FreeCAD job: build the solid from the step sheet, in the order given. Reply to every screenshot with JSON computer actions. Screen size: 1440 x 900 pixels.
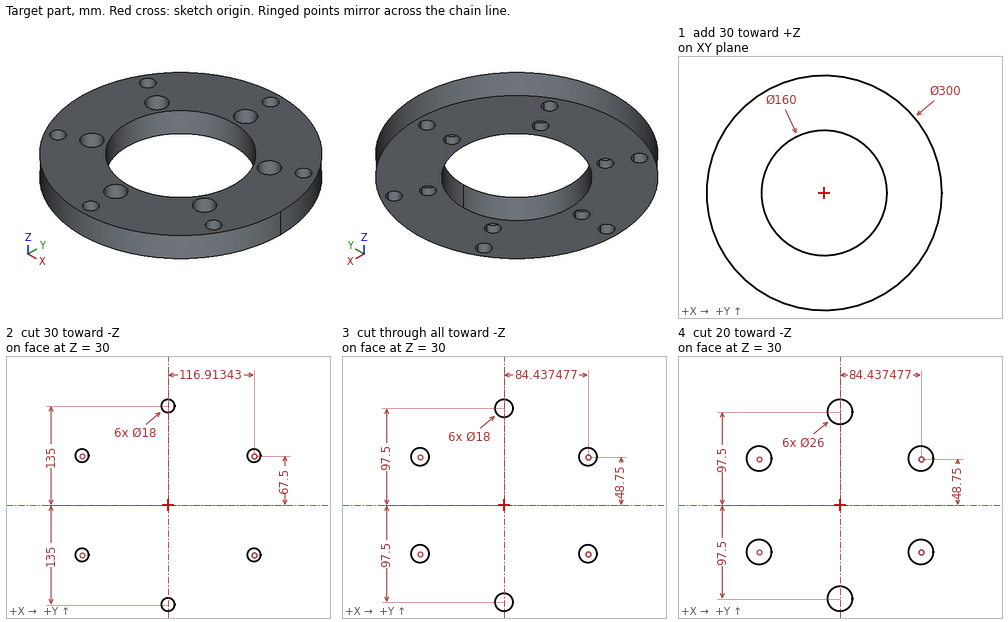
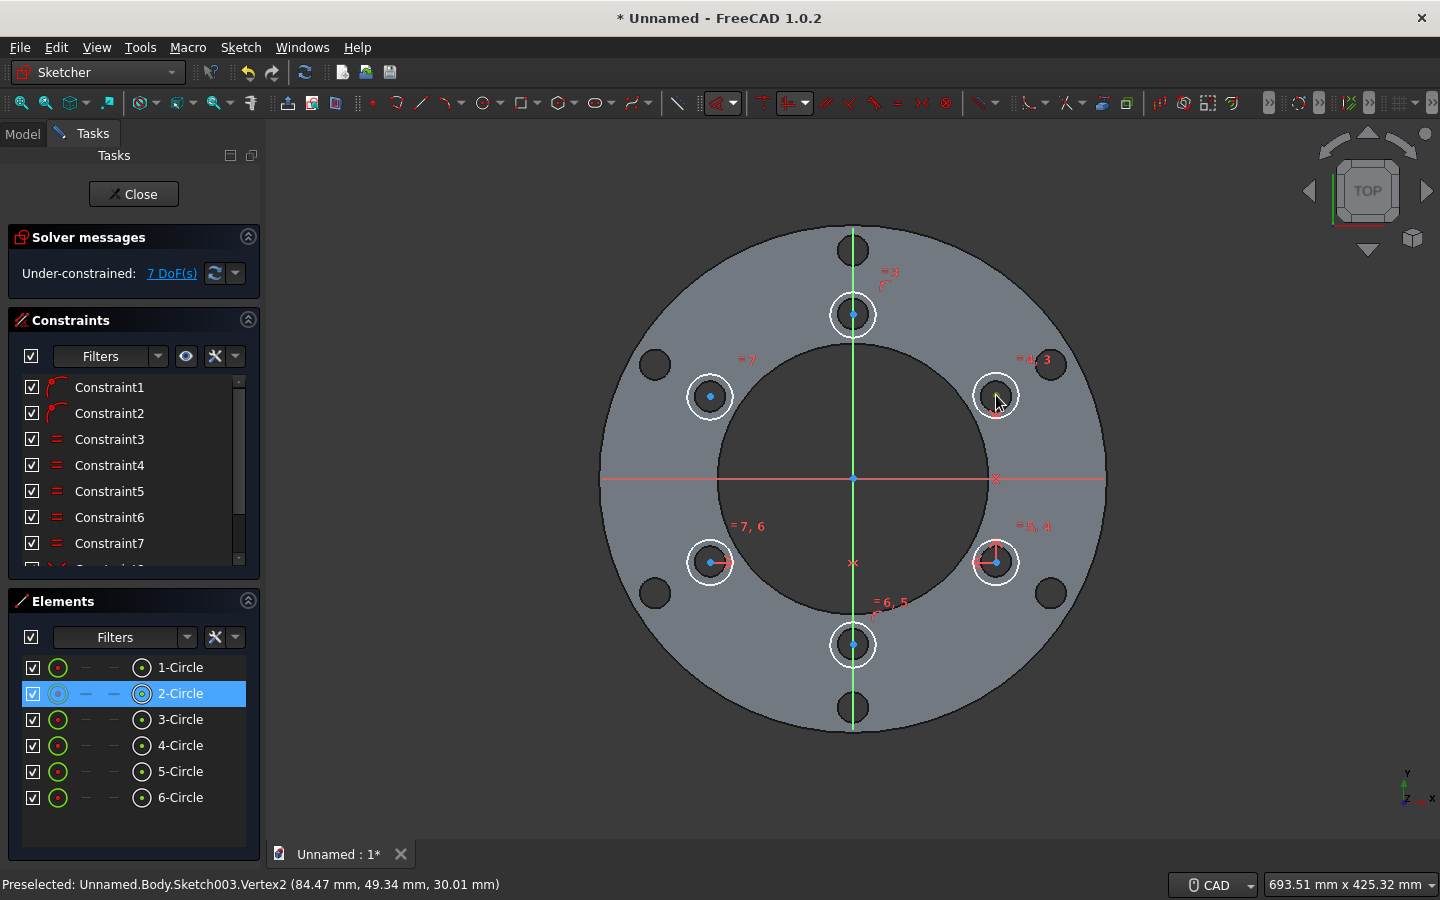
{"action": "left_click", "coordinate": [710, 397]}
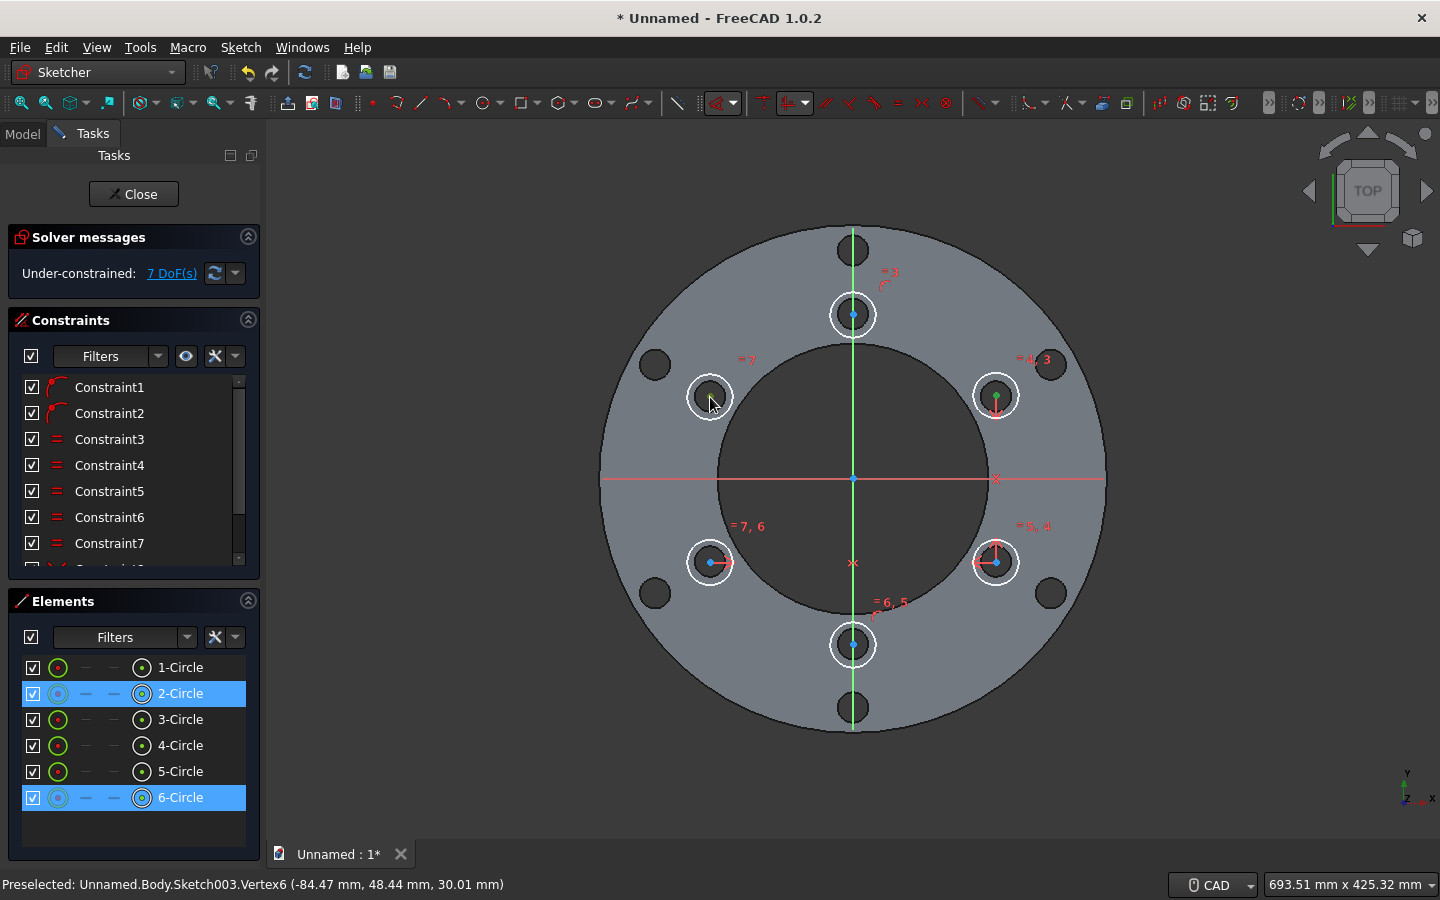
{"action": "left_click", "coordinate": [853, 716]}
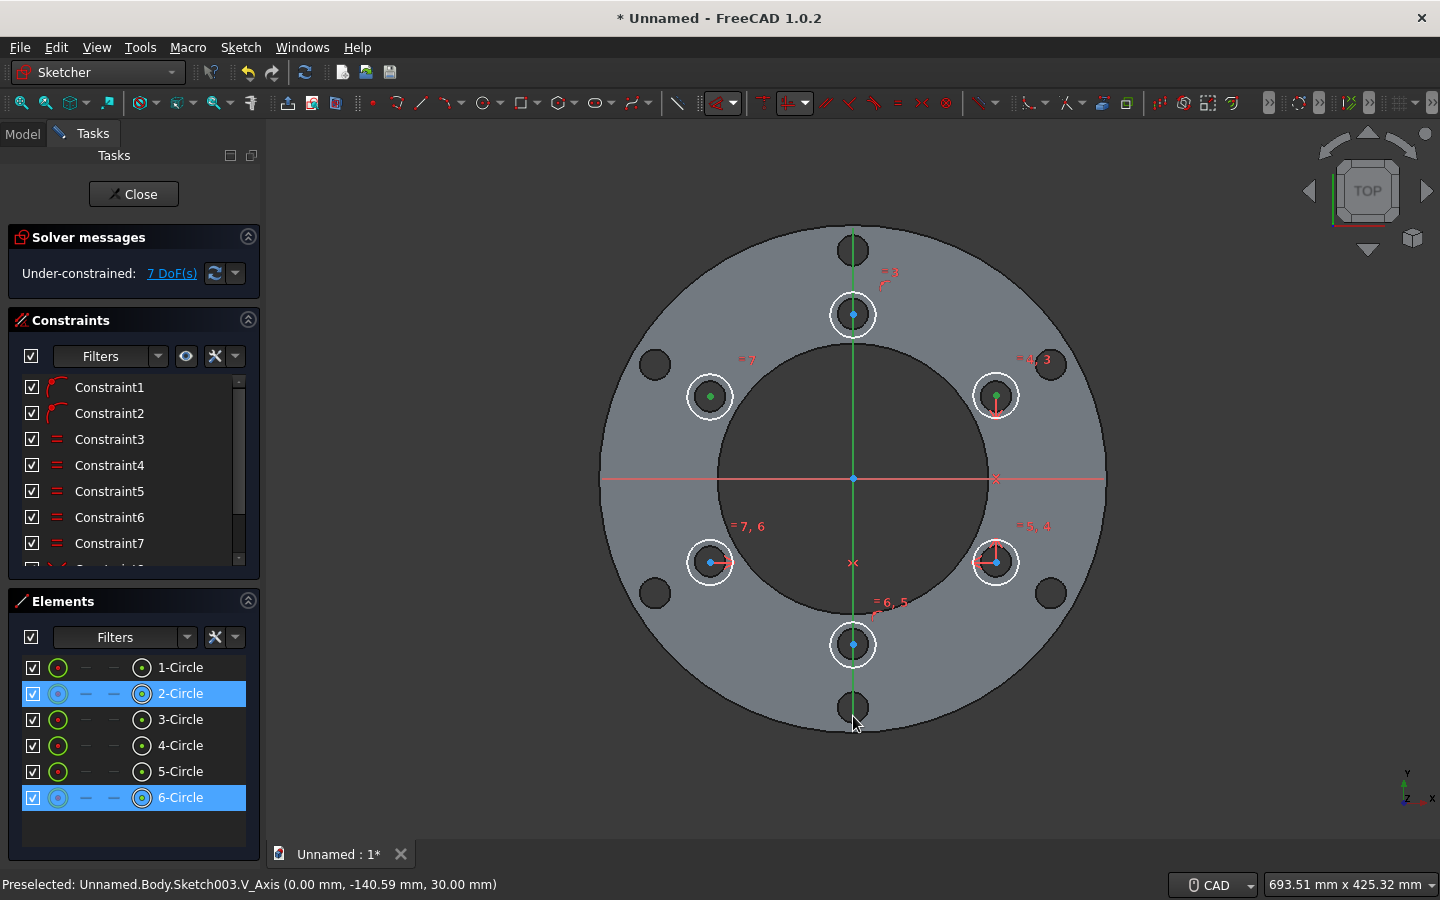
{"action": "key", "text": "s"}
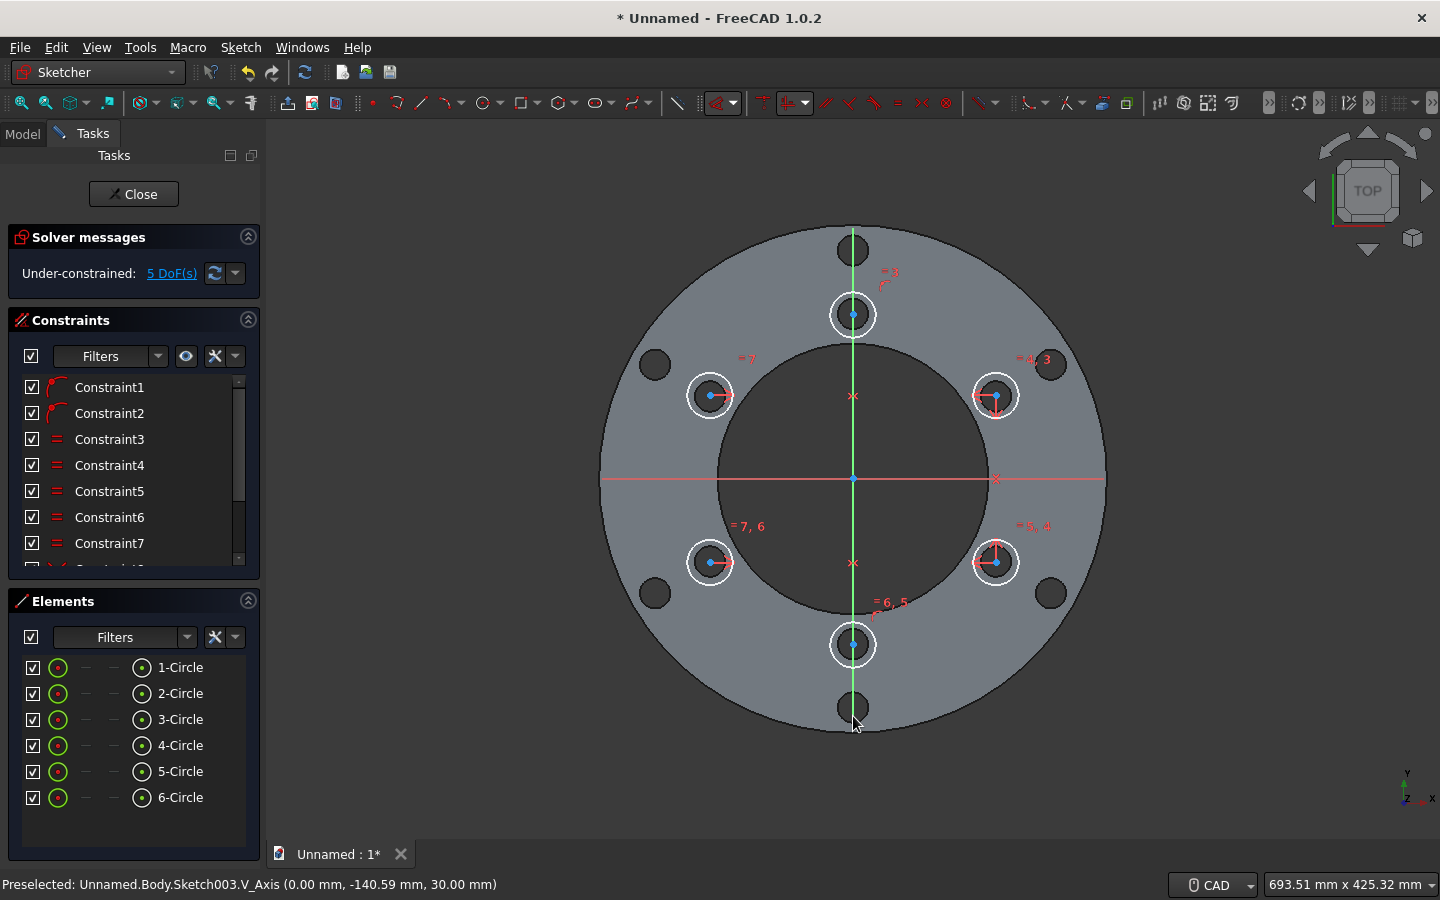
{"action": "left_click", "coordinate": [869, 299]}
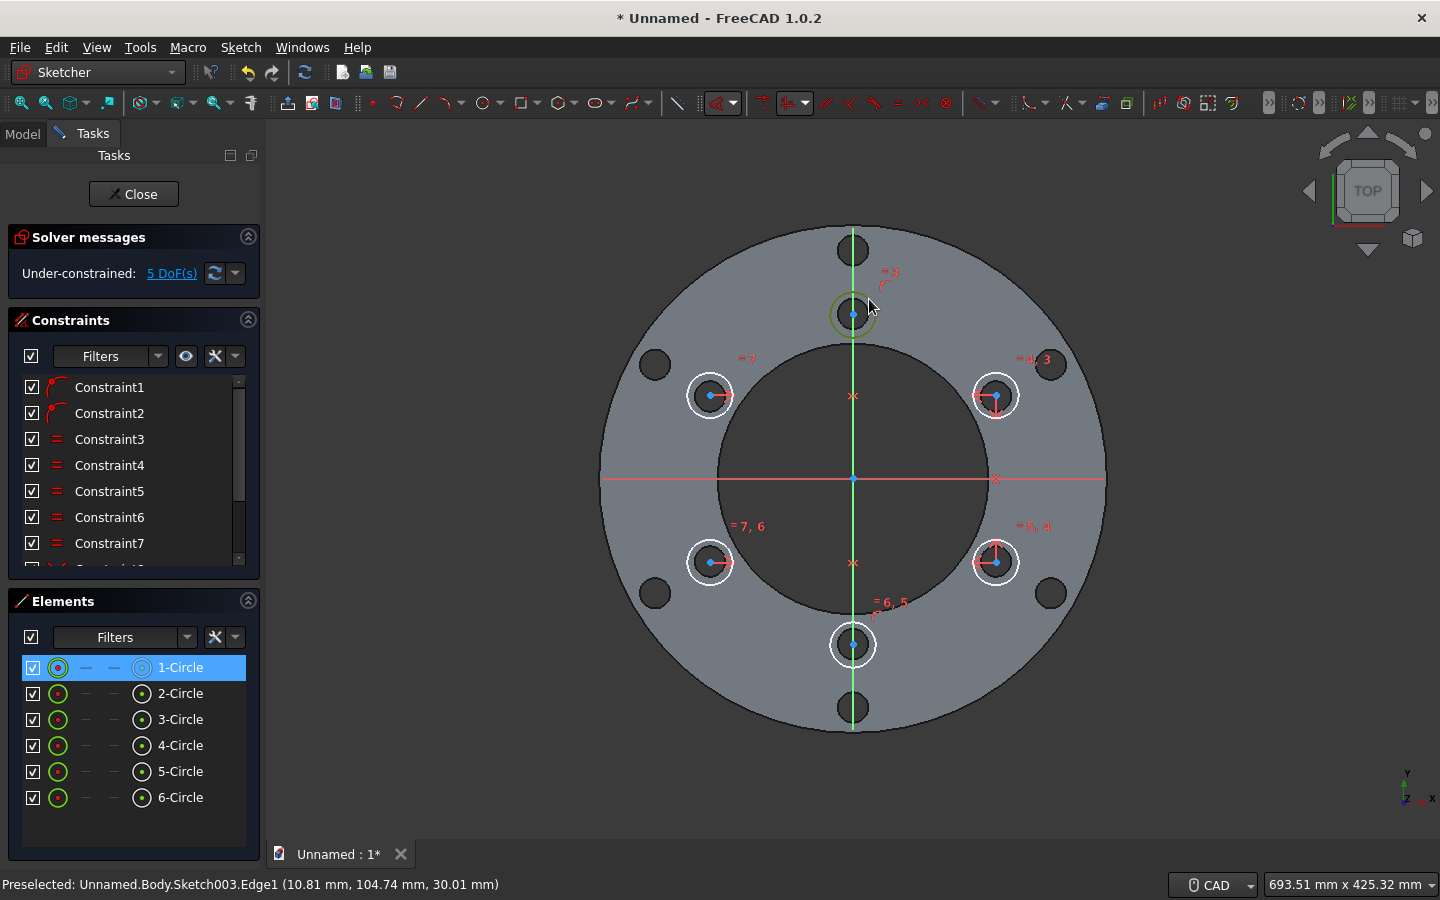
{"action": "key", "text": "k o"}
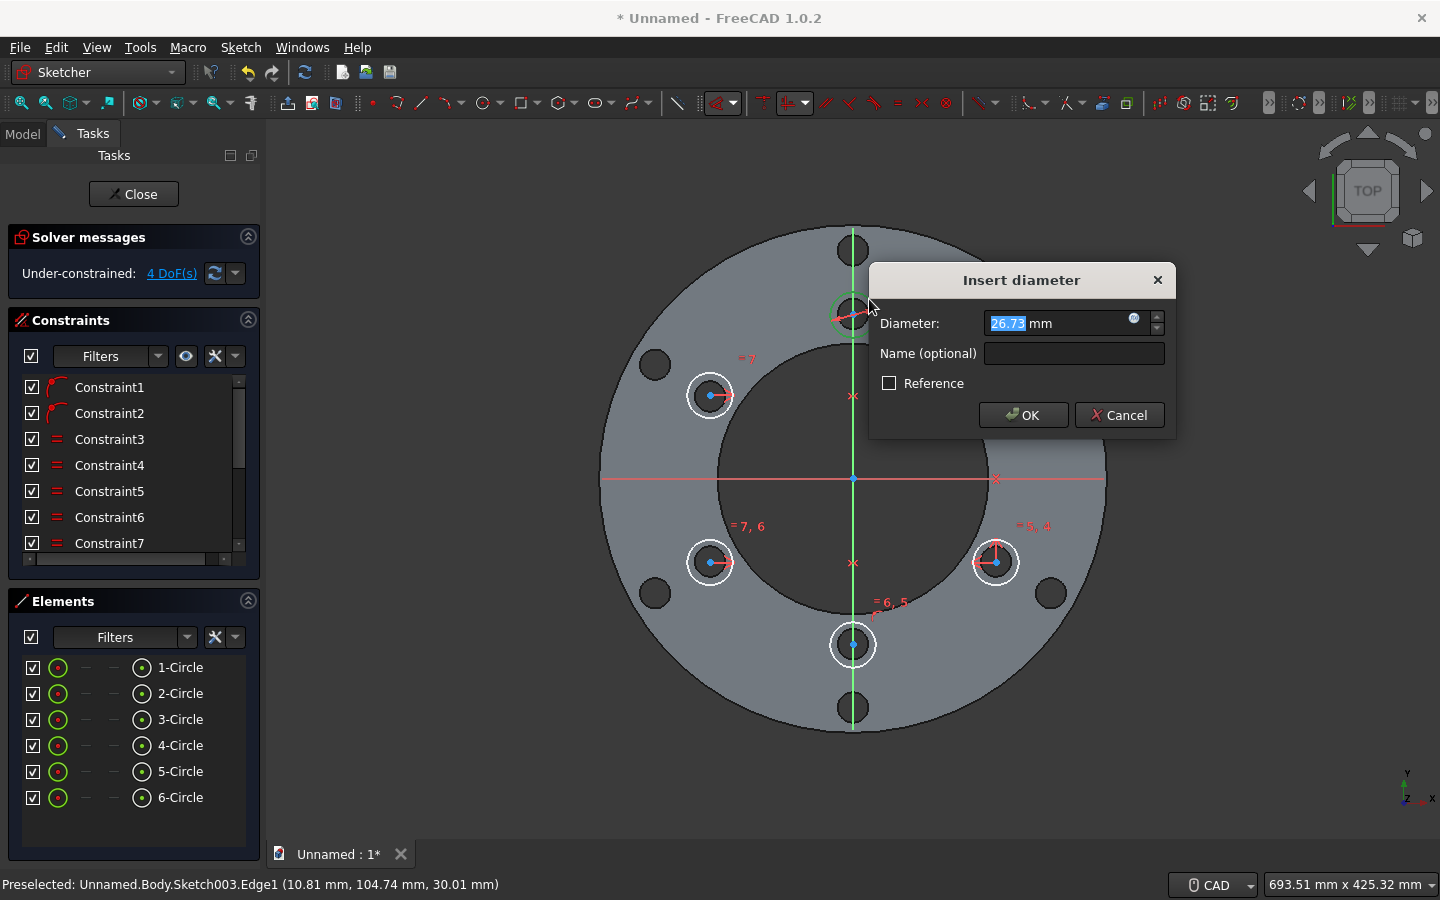
{"action": "type", "text": "26"}
{"action": "key", "text": "Return"}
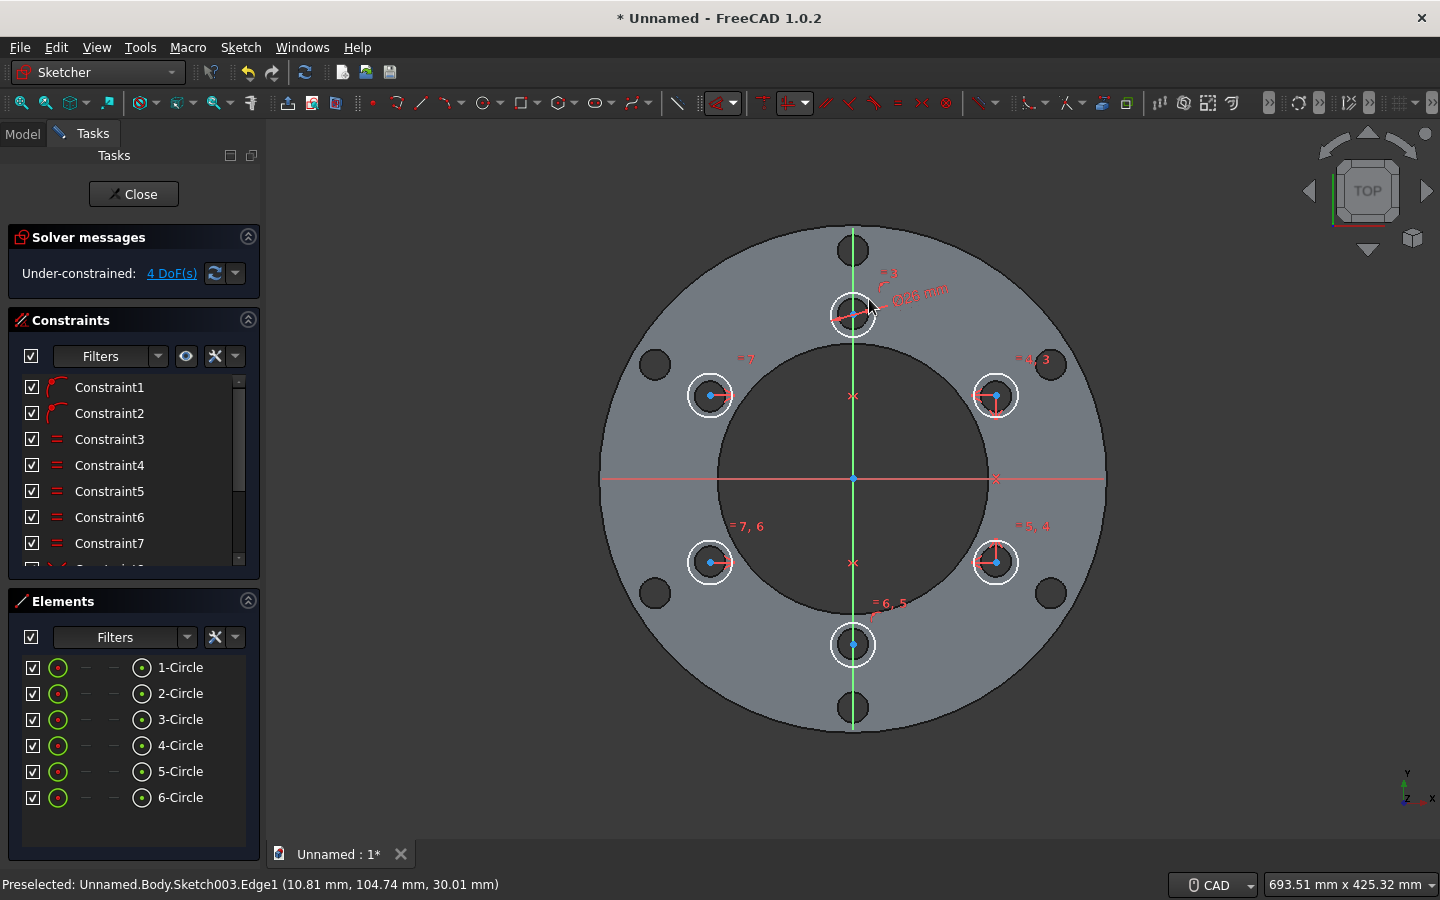
{"action": "left_click", "coordinate": [853, 315]}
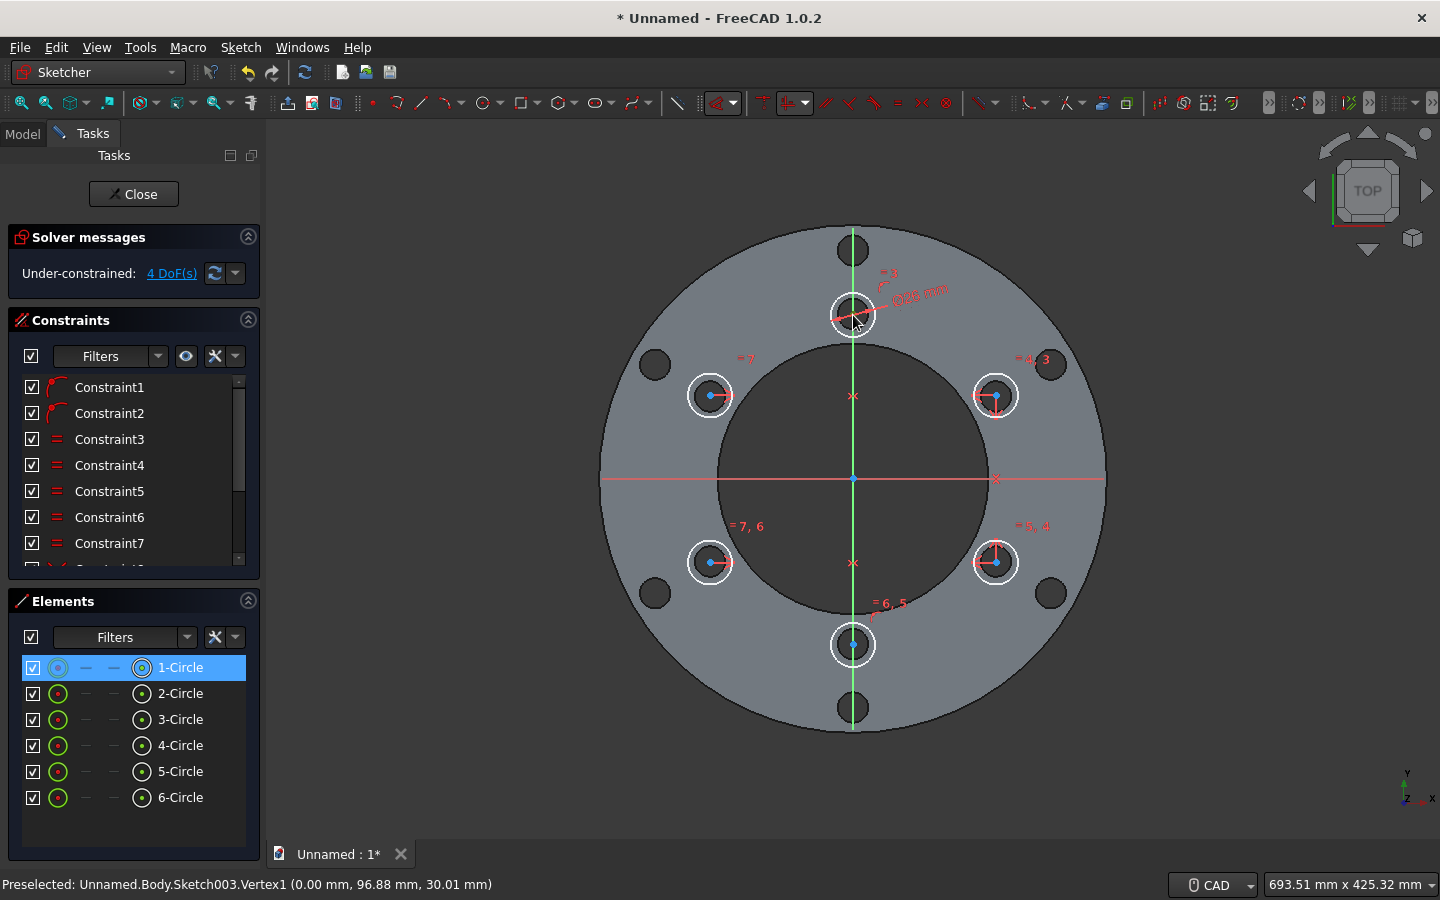
{"action": "key", "text": "i"}